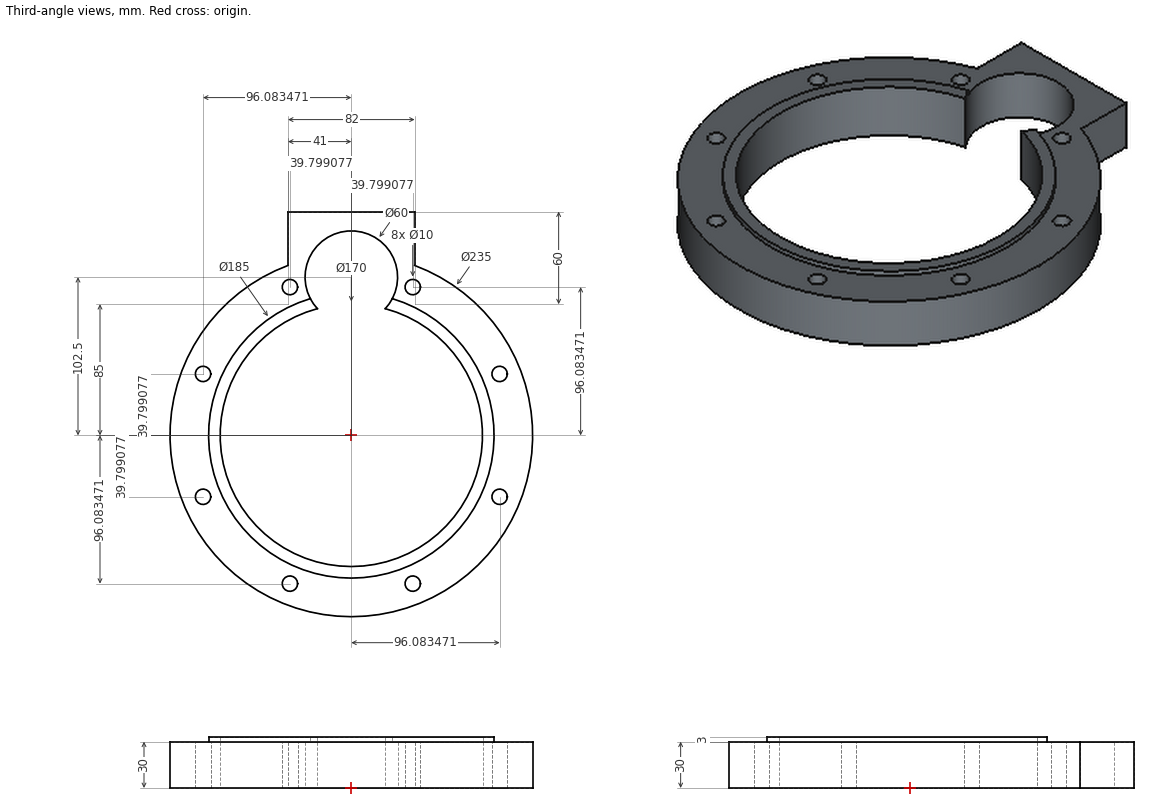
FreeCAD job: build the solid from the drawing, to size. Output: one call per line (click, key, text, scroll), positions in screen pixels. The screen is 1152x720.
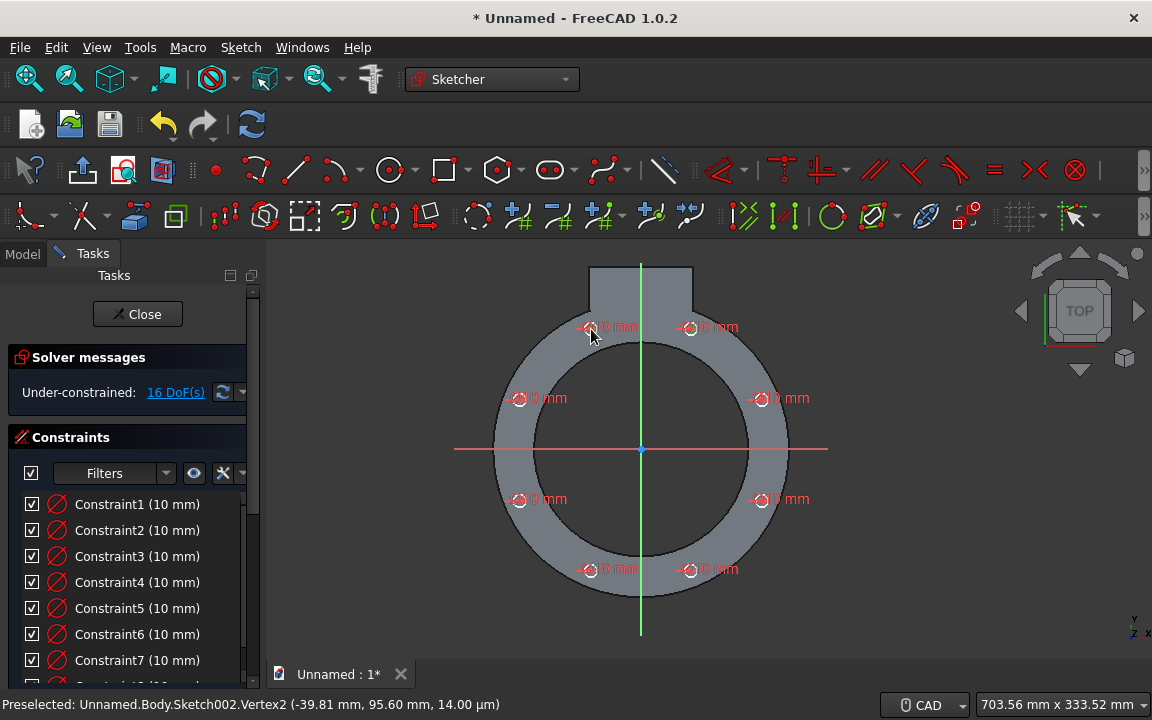
click(848, 170)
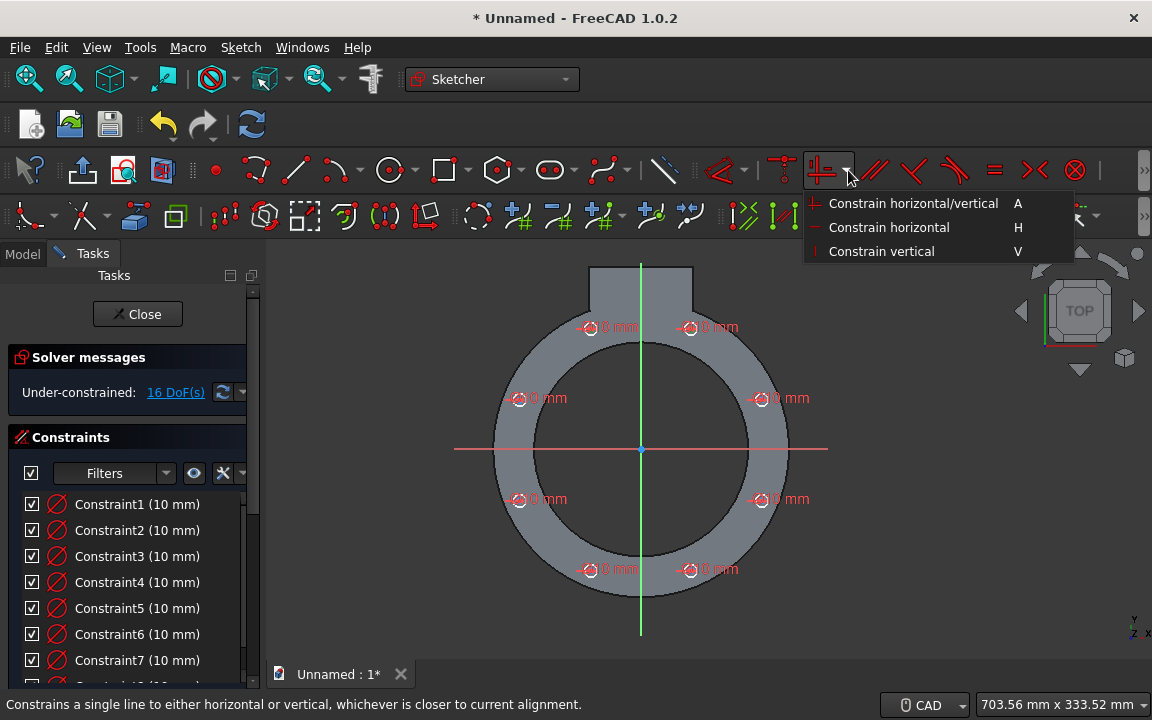
click(939, 227)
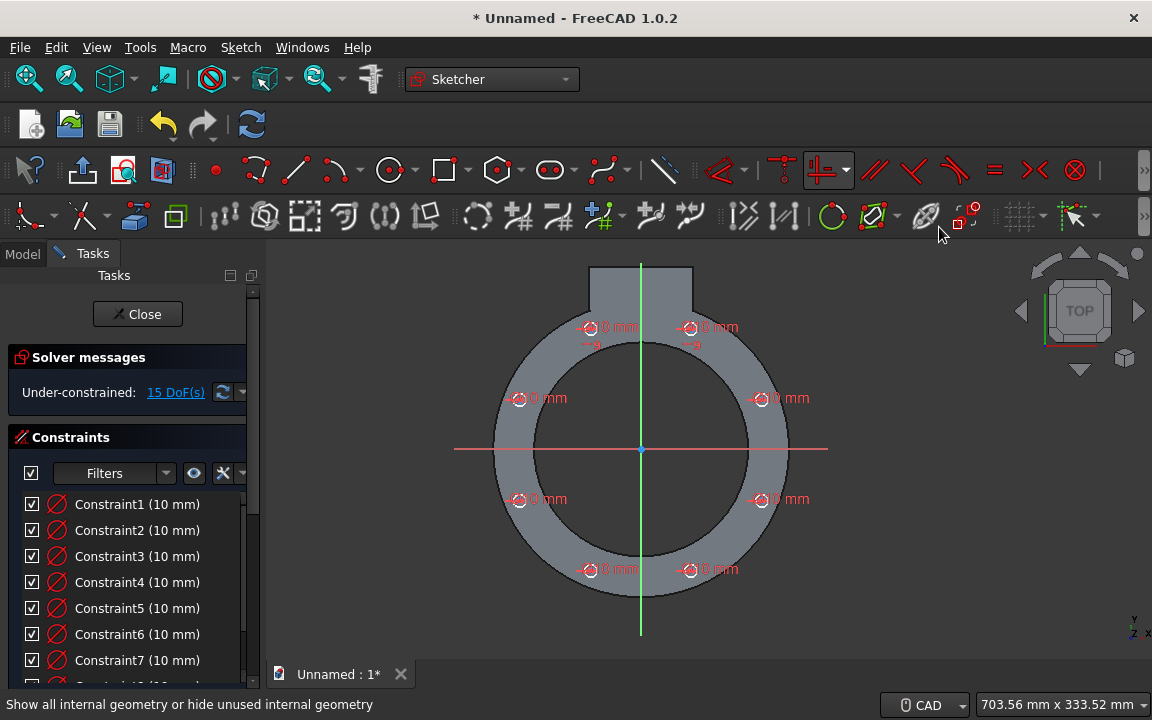
click(520, 400)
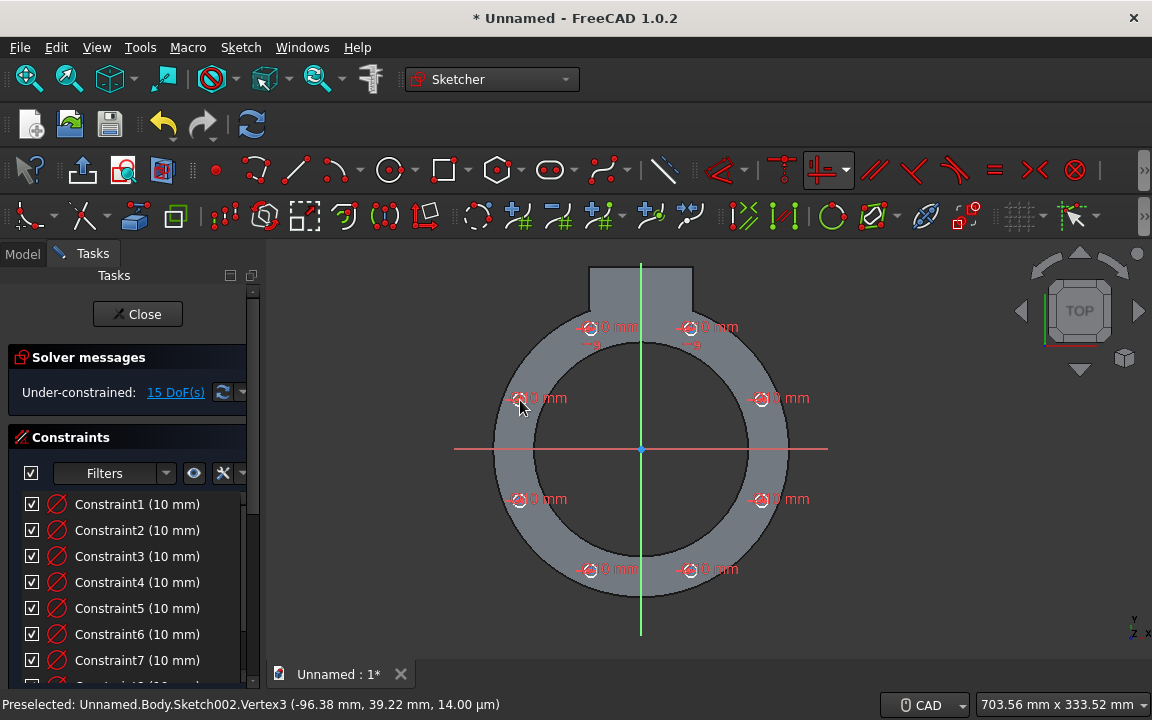
click(520, 501)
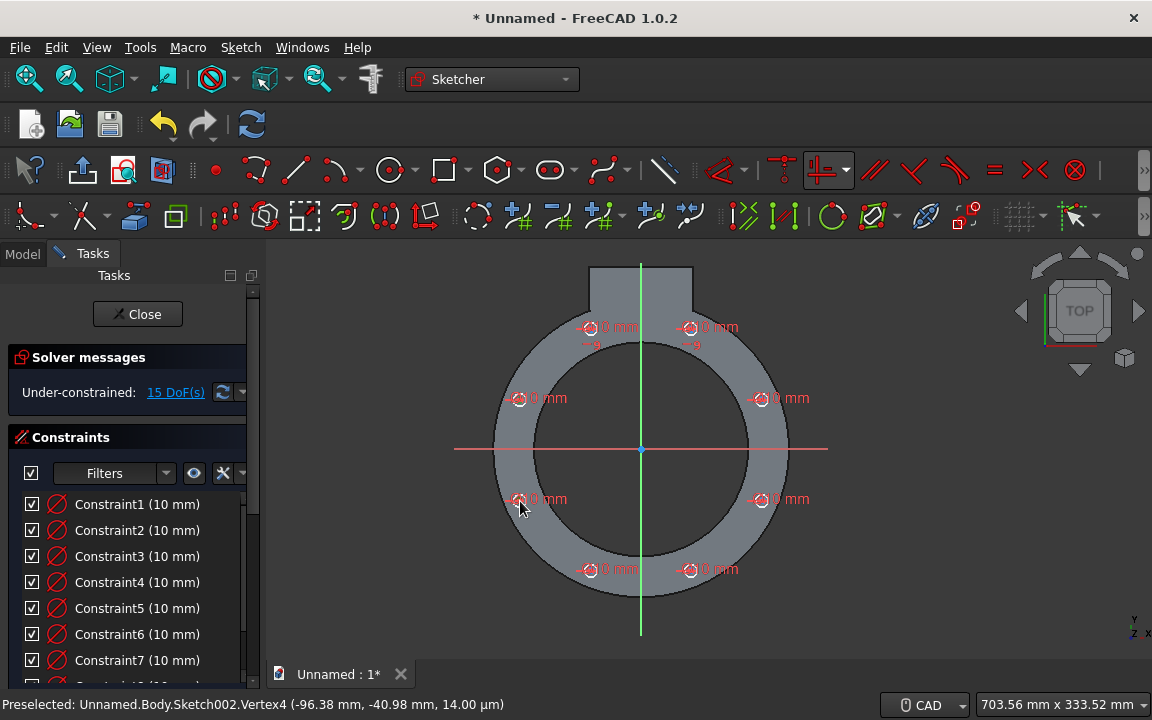
click(848, 170)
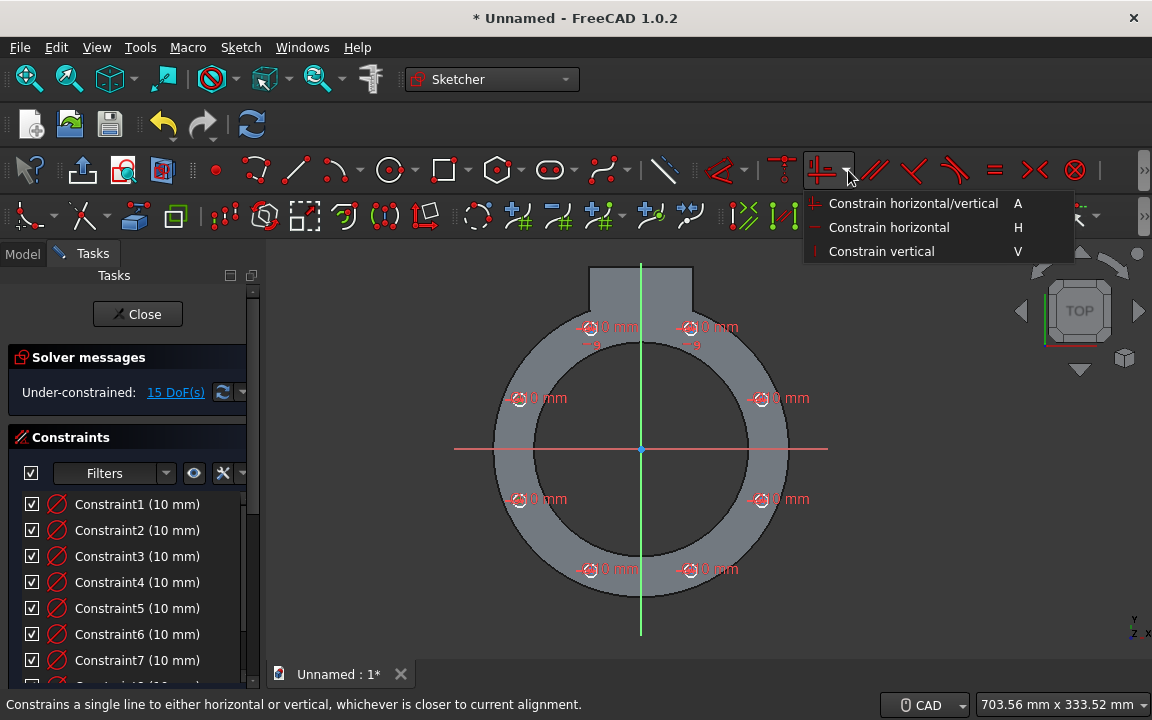
click(939, 251)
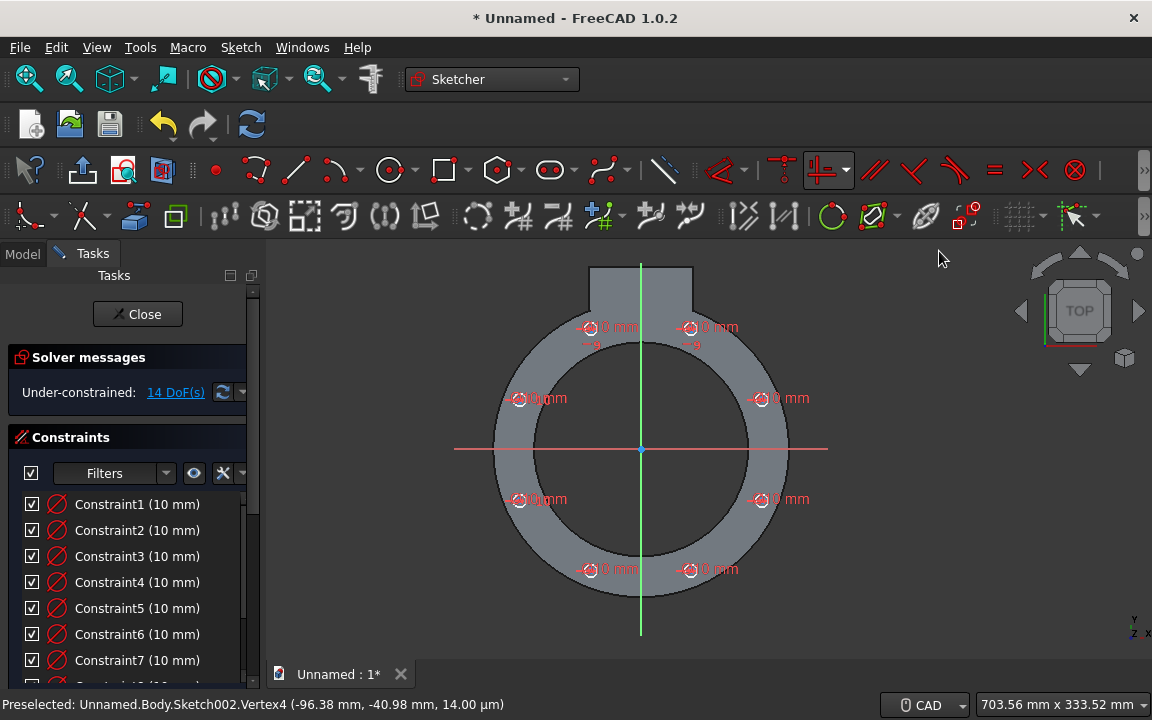
click(591, 329)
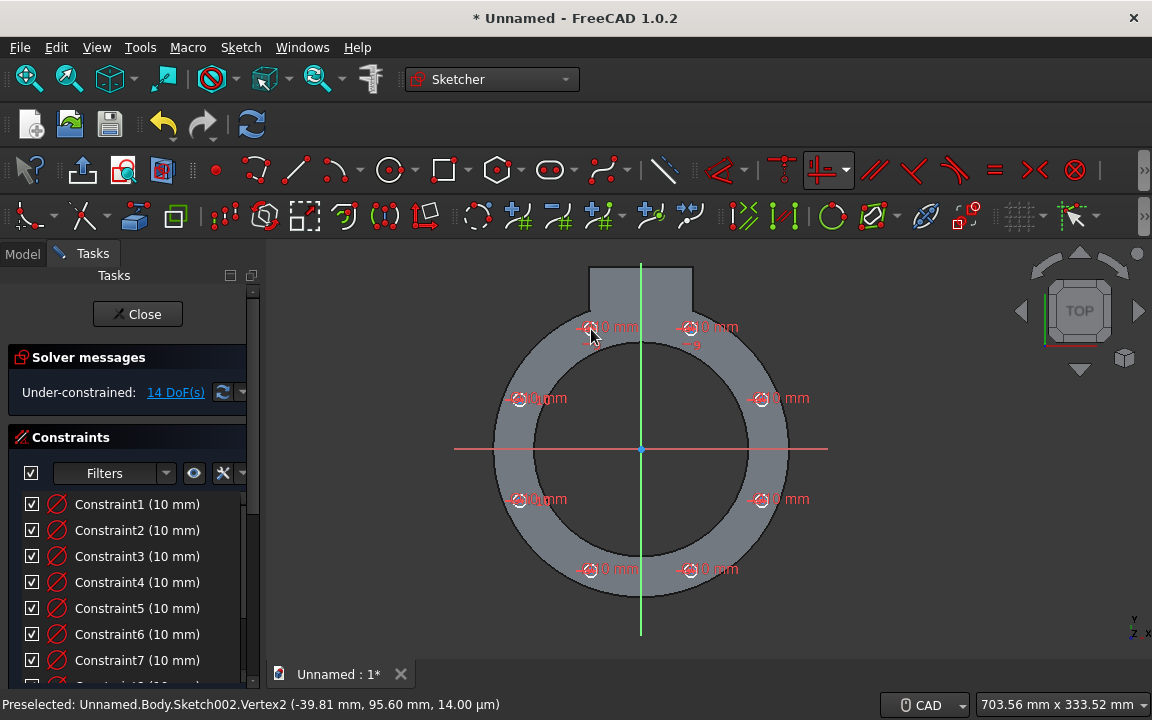
click(591, 571)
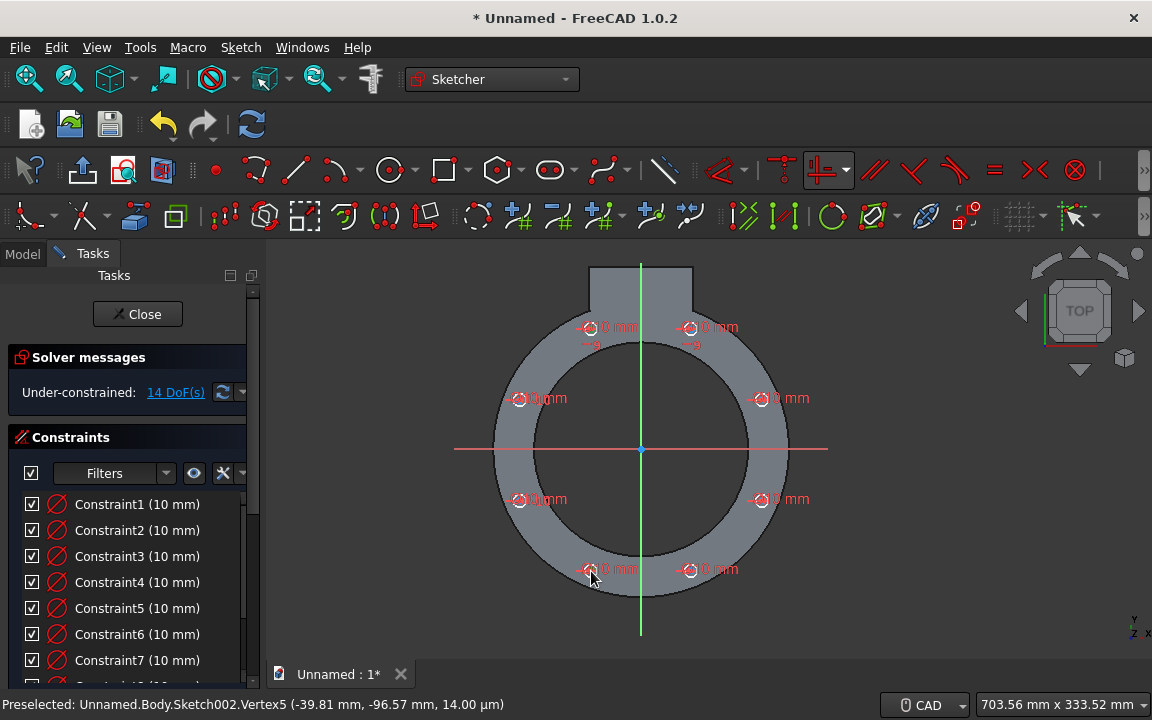
key(v)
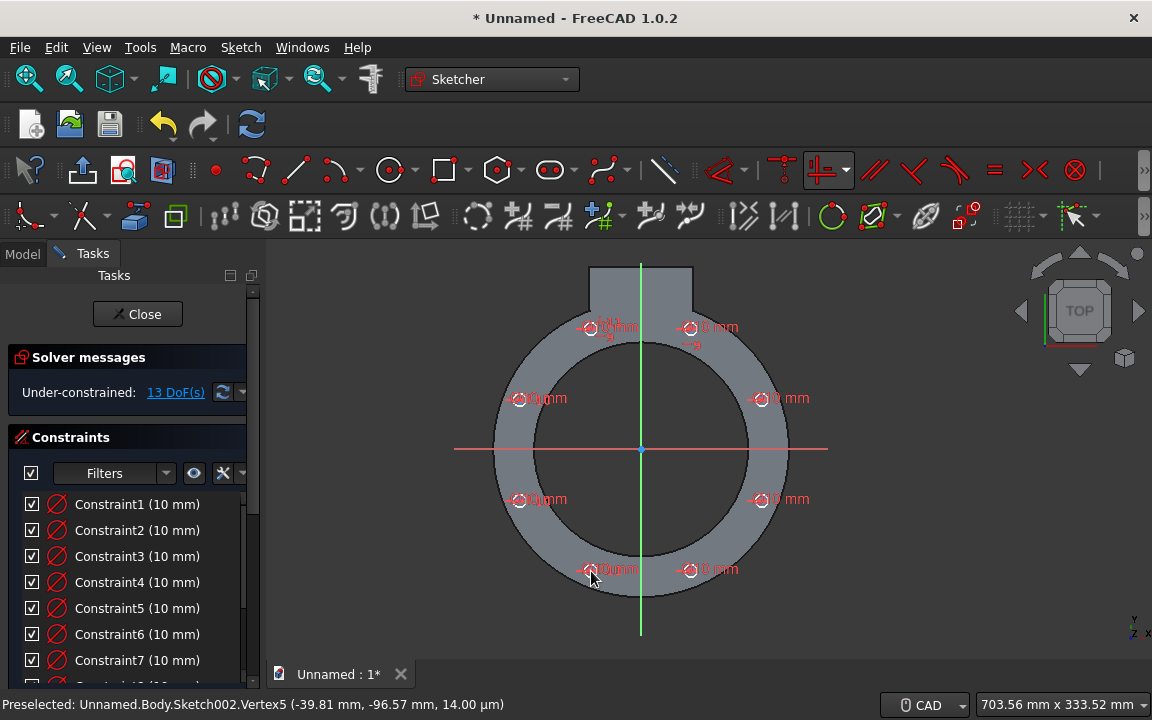
click(691, 329)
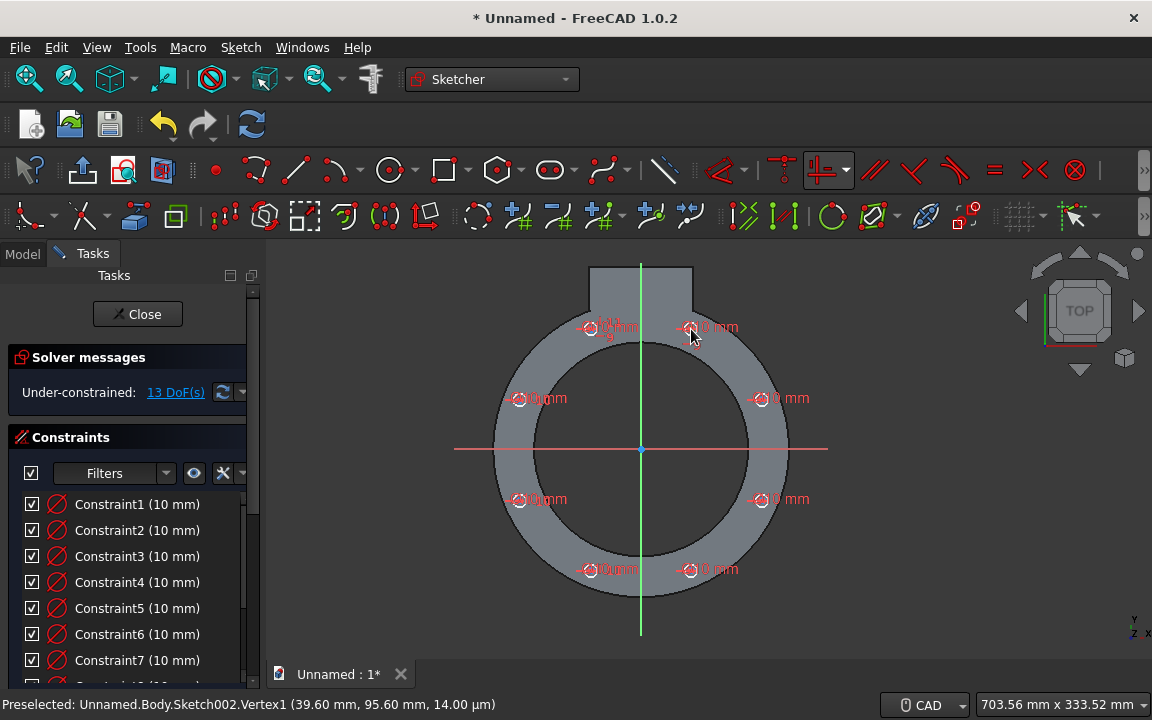
click(691, 571)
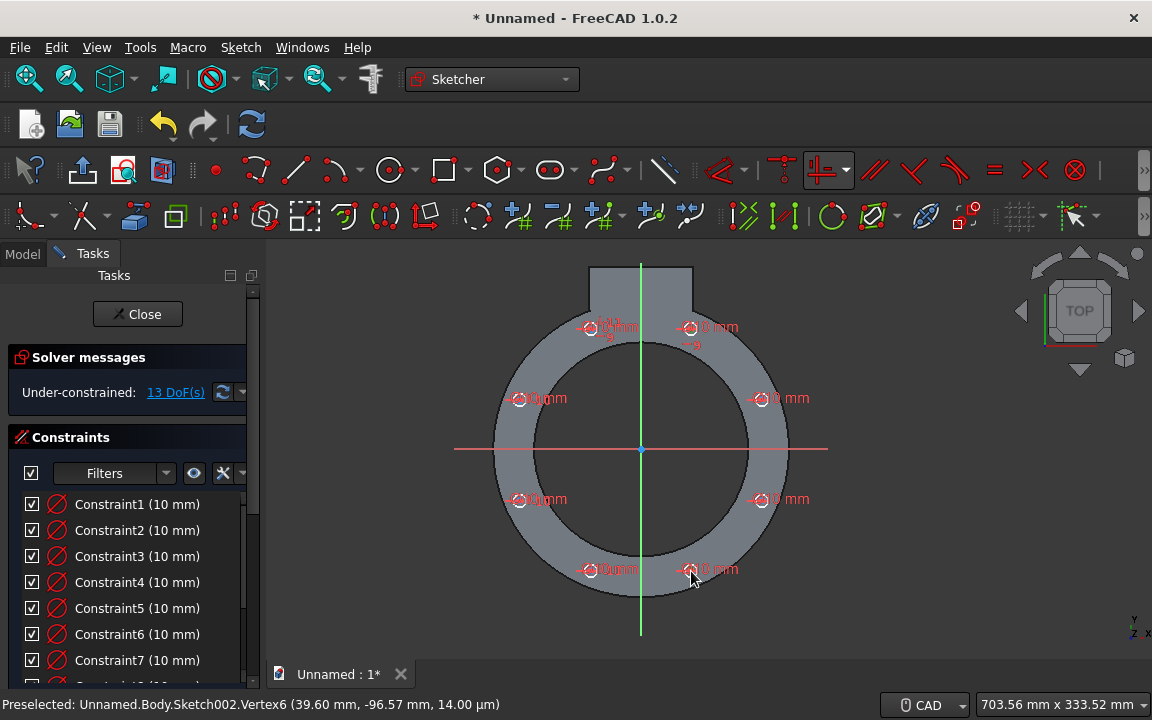
key(v)